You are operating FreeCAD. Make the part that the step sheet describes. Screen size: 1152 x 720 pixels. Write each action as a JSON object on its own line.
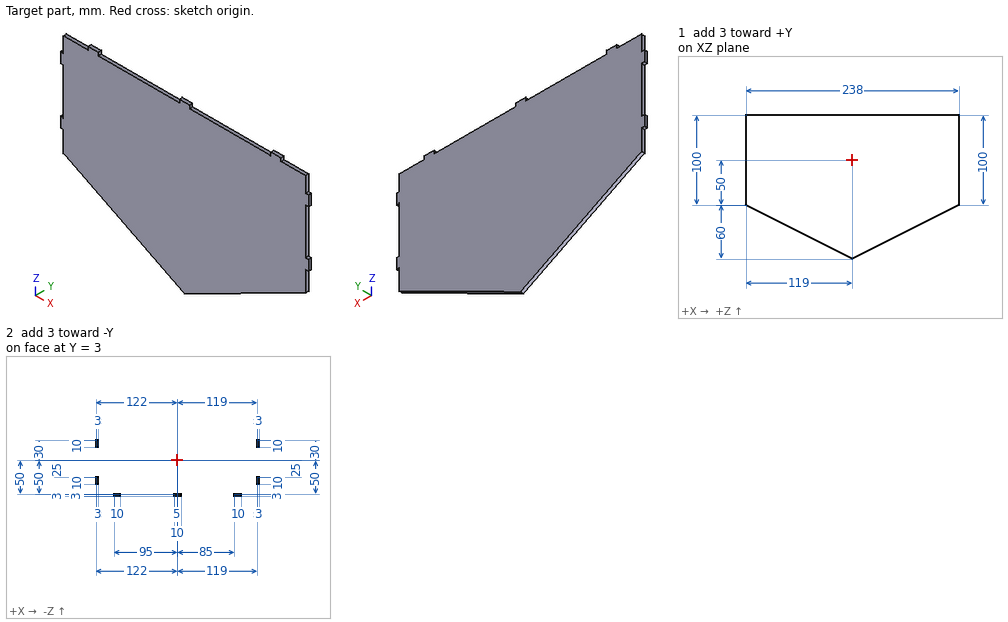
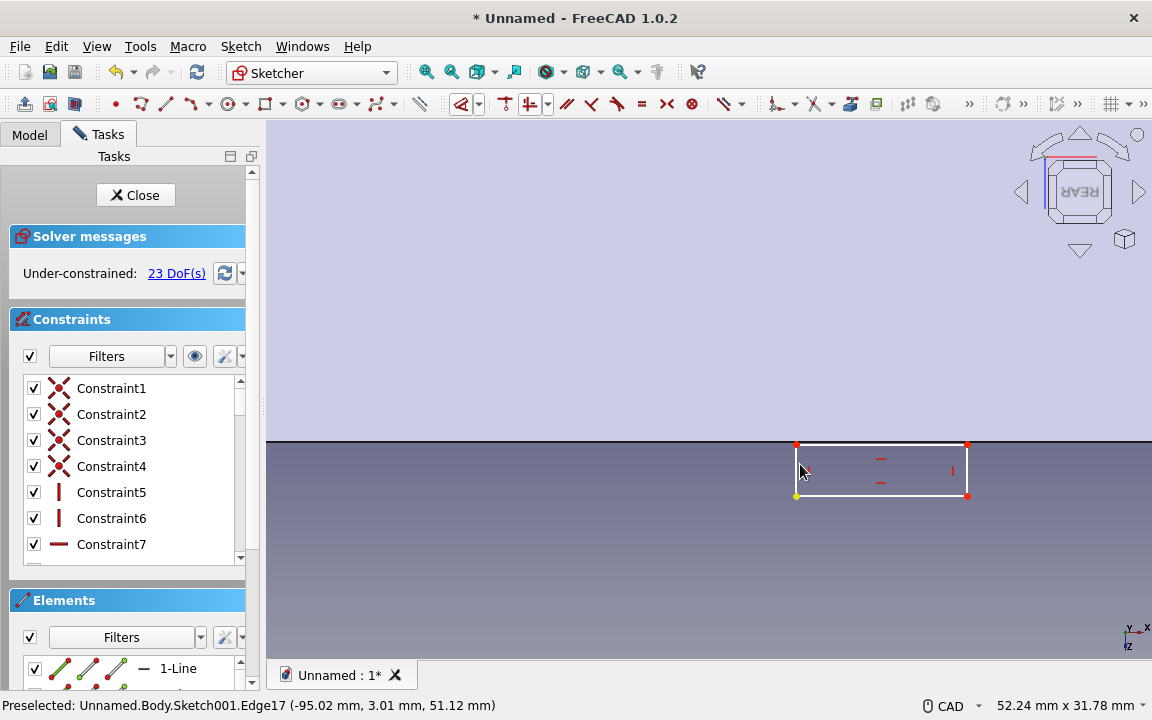
{"action": "left_click", "coordinate": [796, 460]}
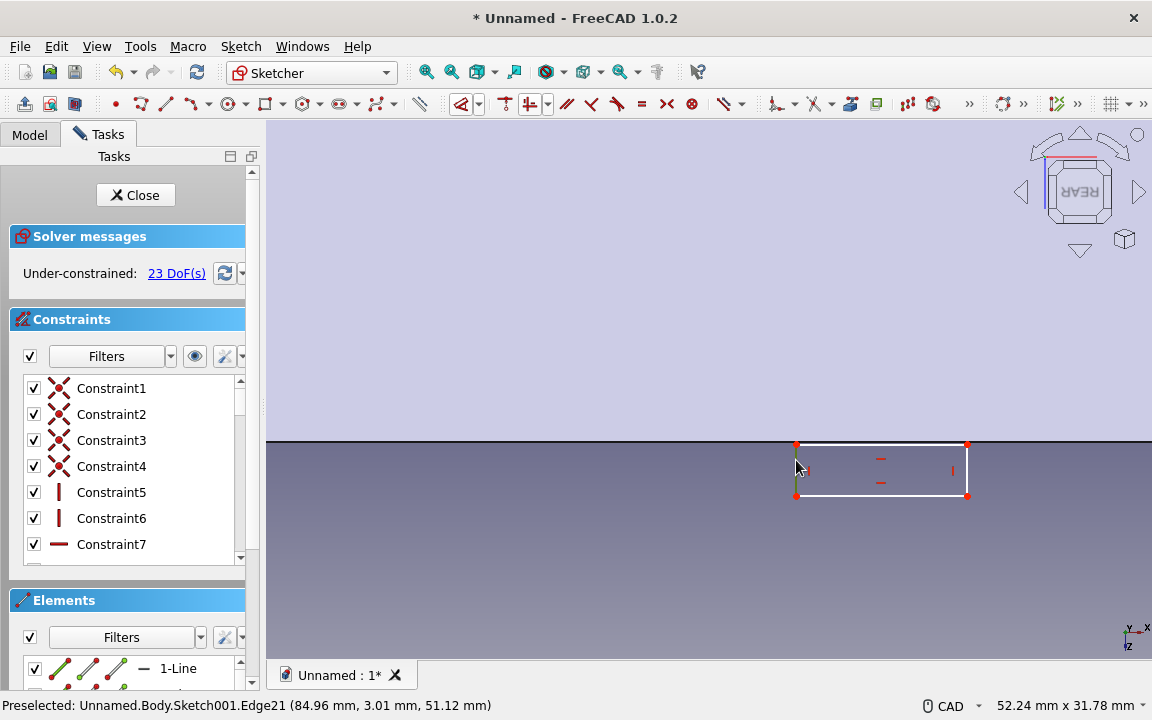
{"action": "left_click", "coordinate": [478, 104]}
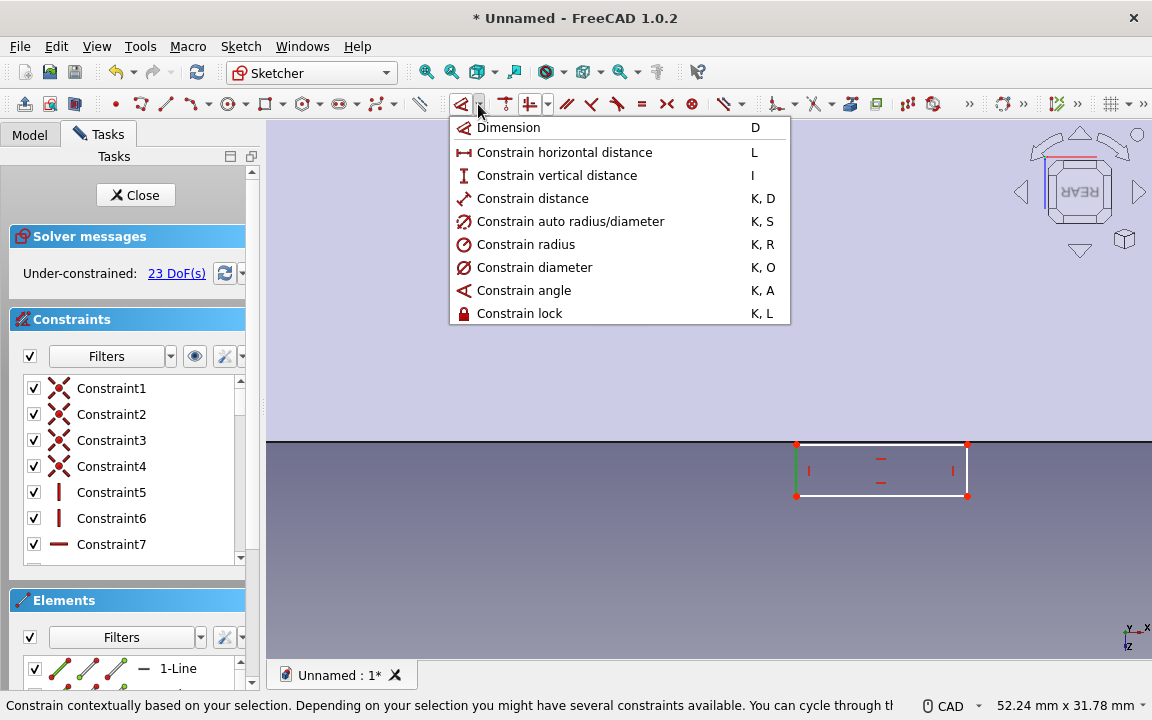
{"action": "left_click", "coordinate": [620, 176]}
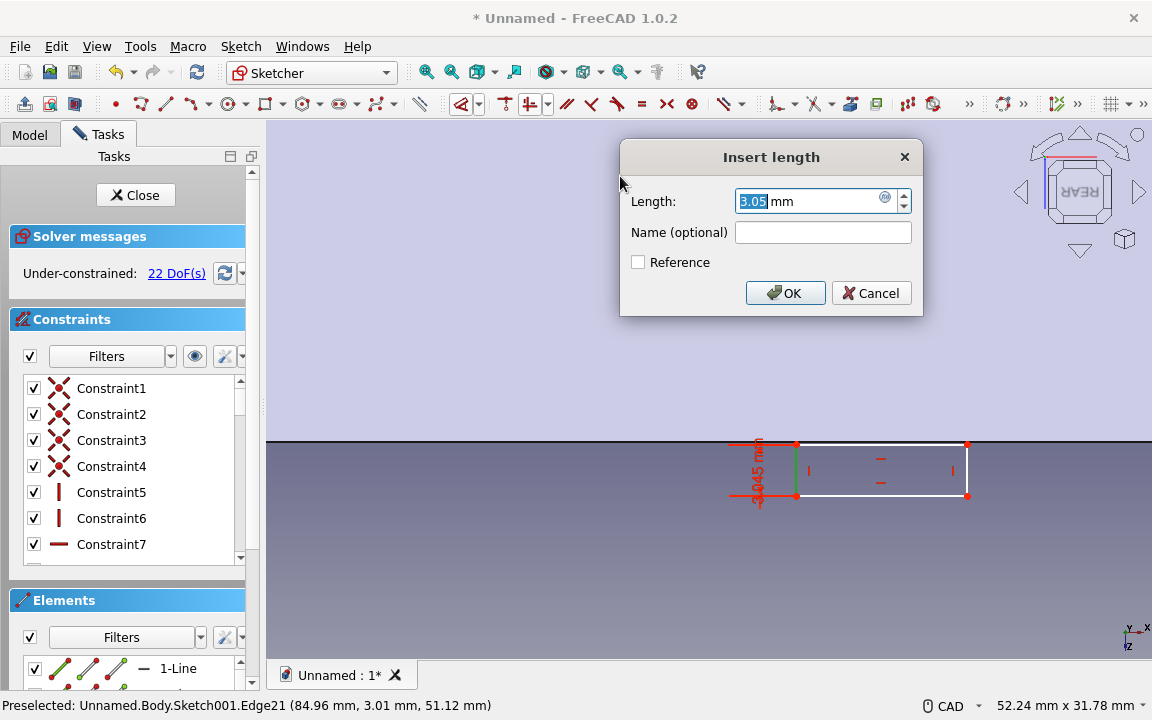
{"action": "type", "text": "3"}
{"action": "key", "text": "Return"}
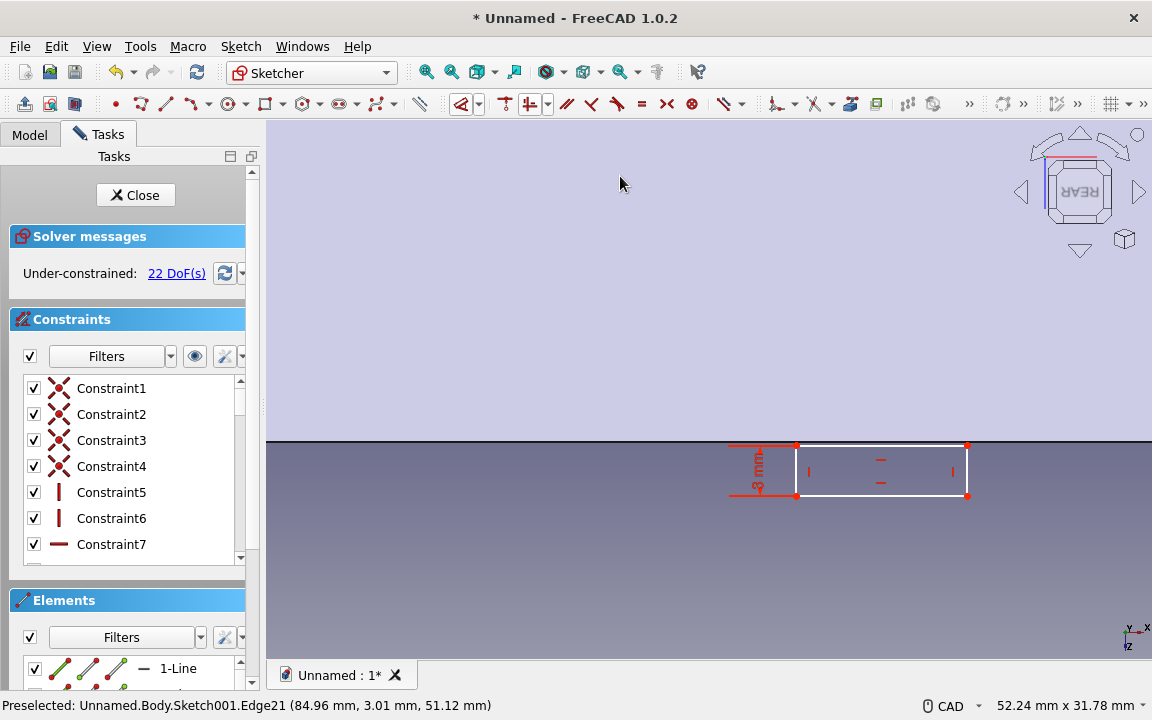
{"action": "scroll", "coordinate": [801, 464], "scroll_direction": "down", "scroll_amount": 11}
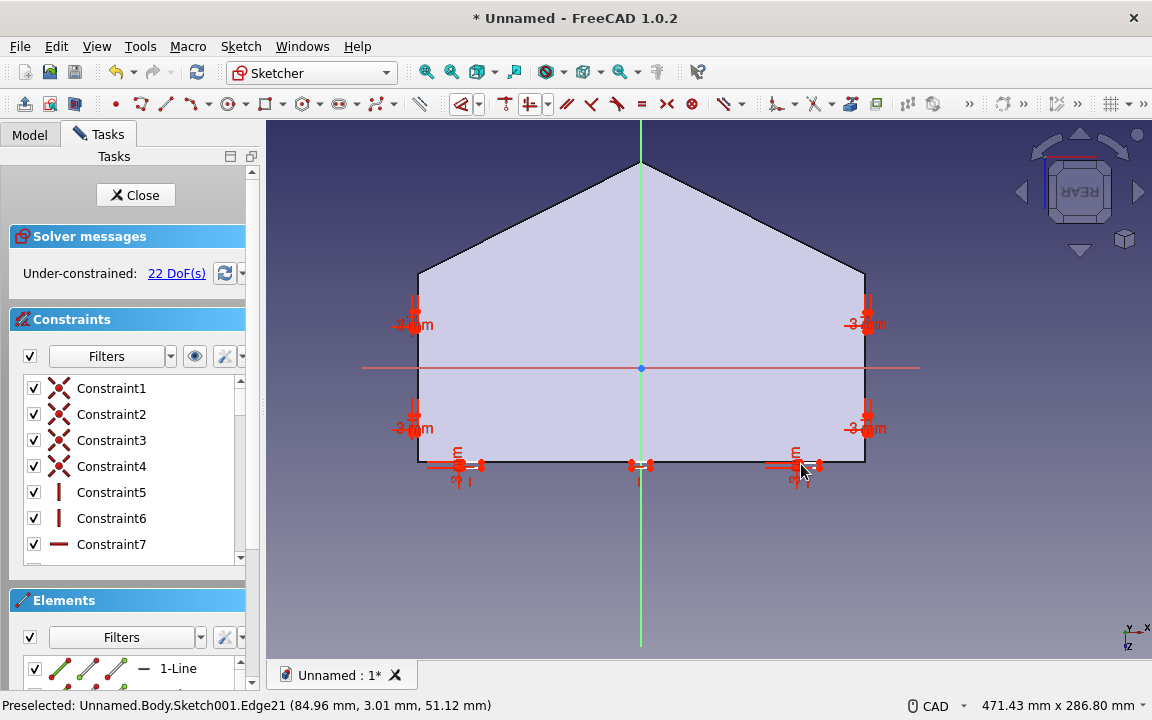
{"action": "scroll", "coordinate": [632, 464], "scroll_direction": "up", "scroll_amount": 11}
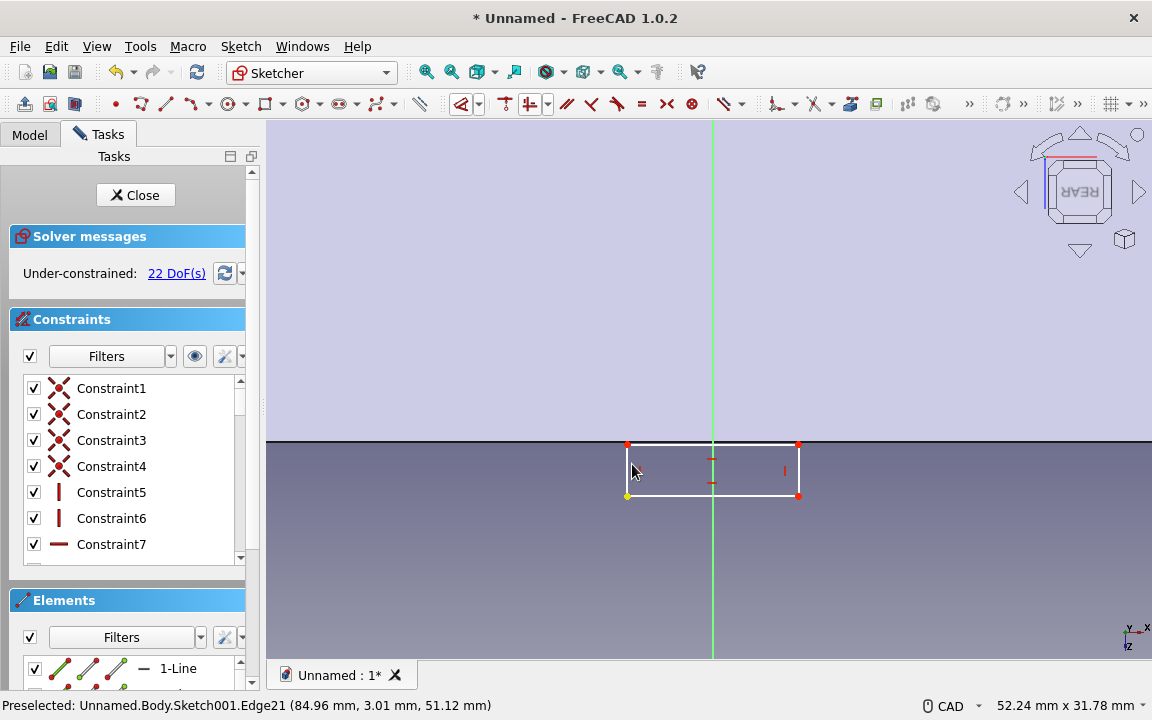
{"action": "left_click", "coordinate": [627, 460]}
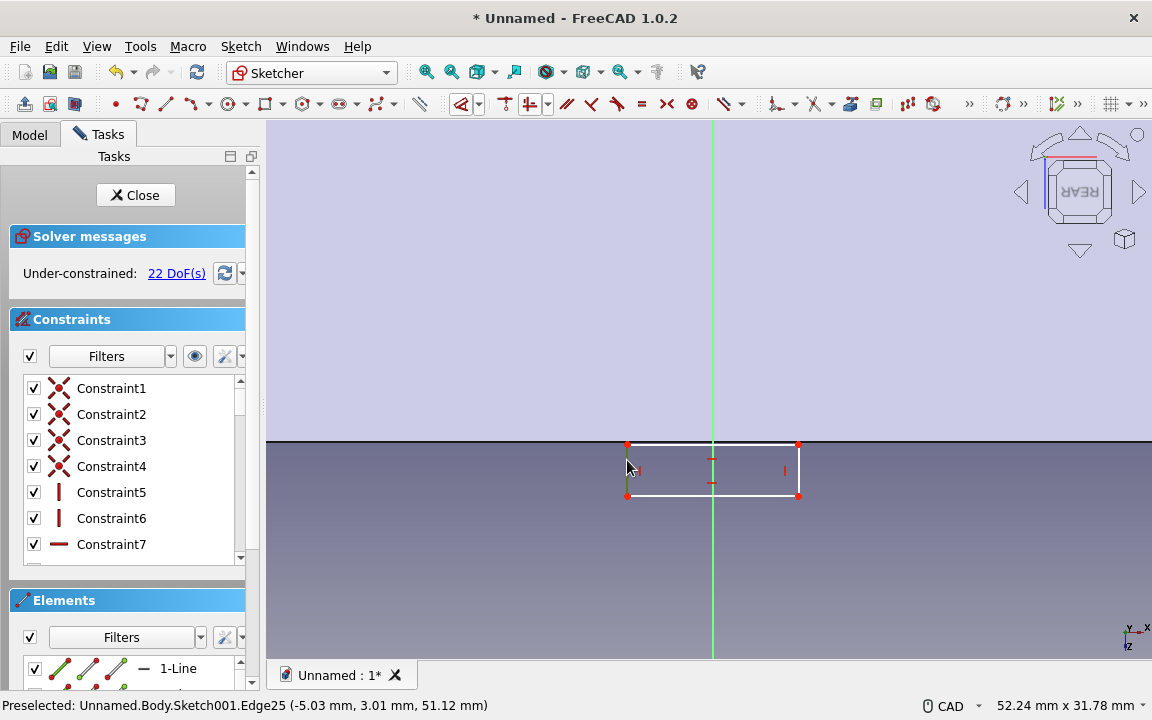
{"action": "key", "text": "i"}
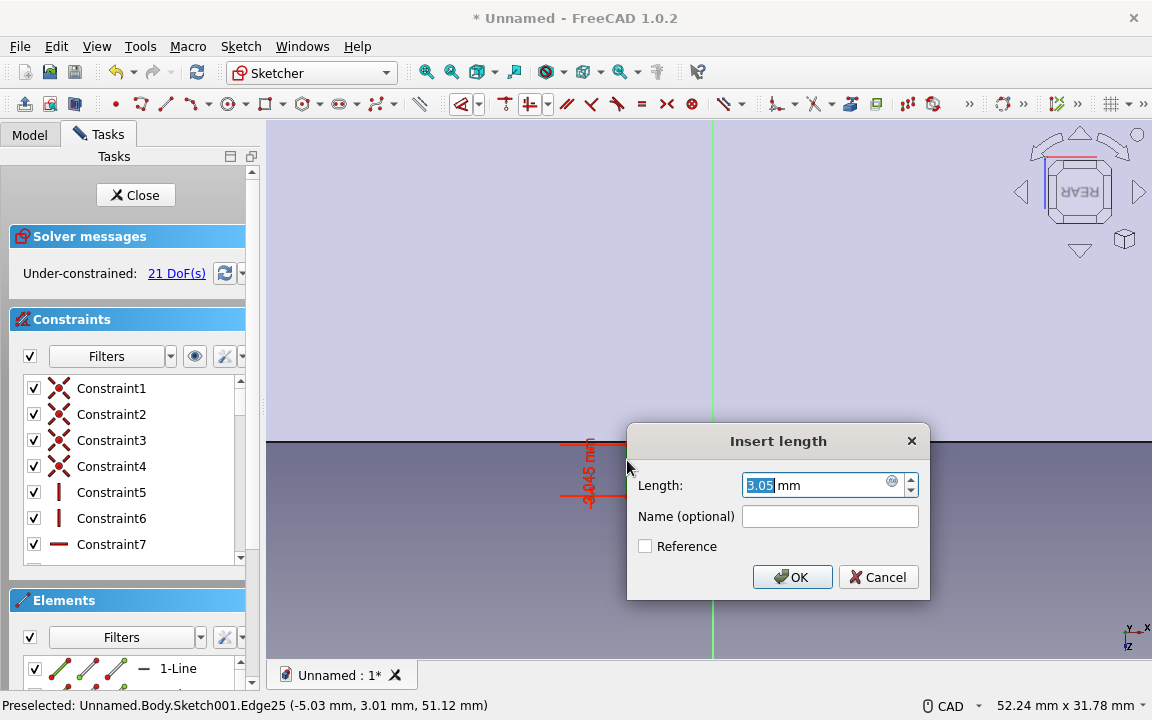
{"action": "type", "text": "3"}
{"action": "key", "text": "Return"}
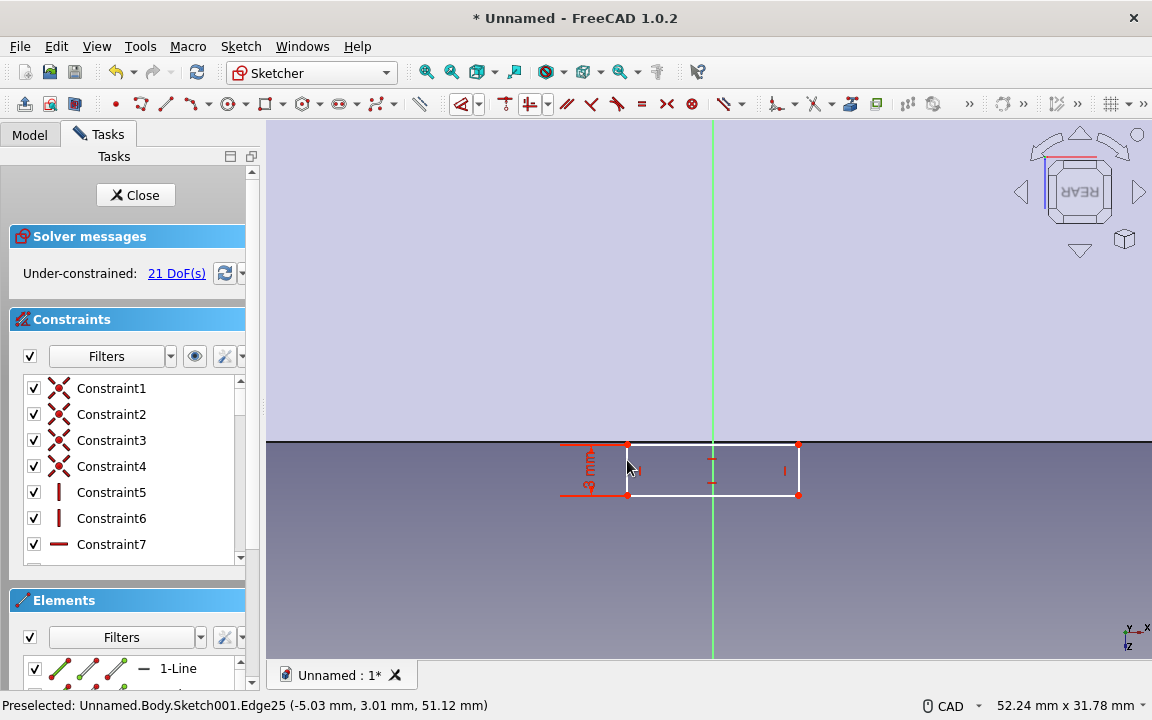
{"action": "scroll", "coordinate": [632, 464], "scroll_direction": "down", "scroll_amount": 11}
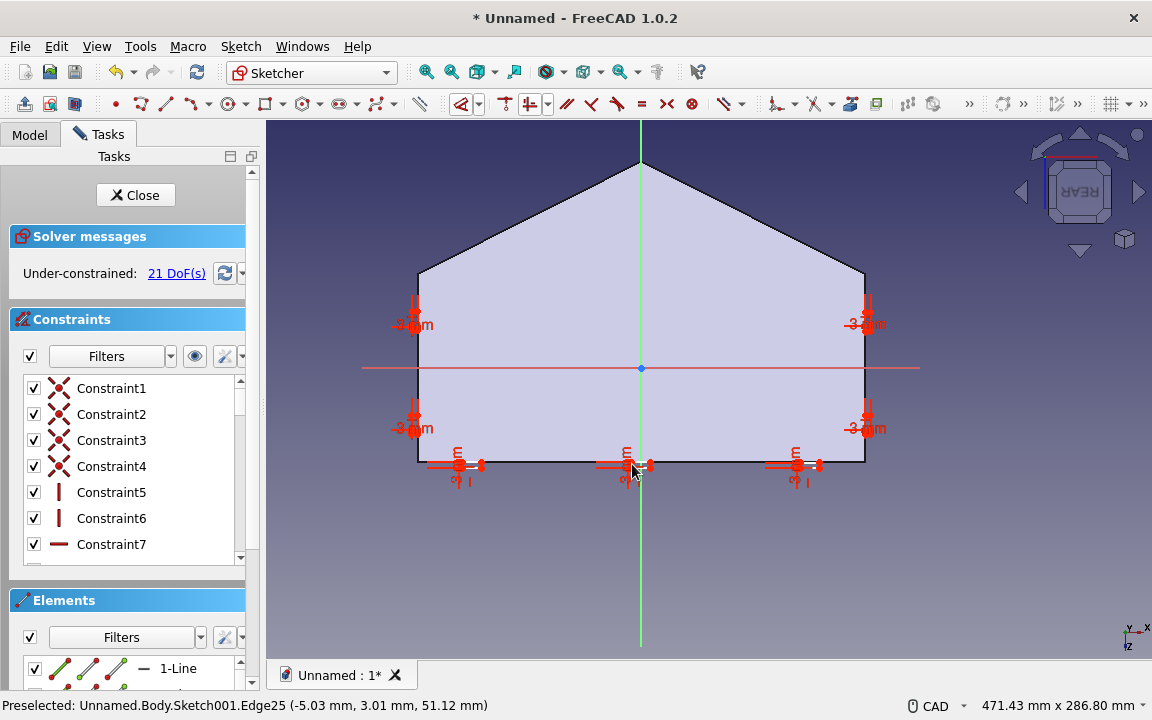
{"action": "scroll", "coordinate": [865, 318], "scroll_direction": "up", "scroll_amount": 5}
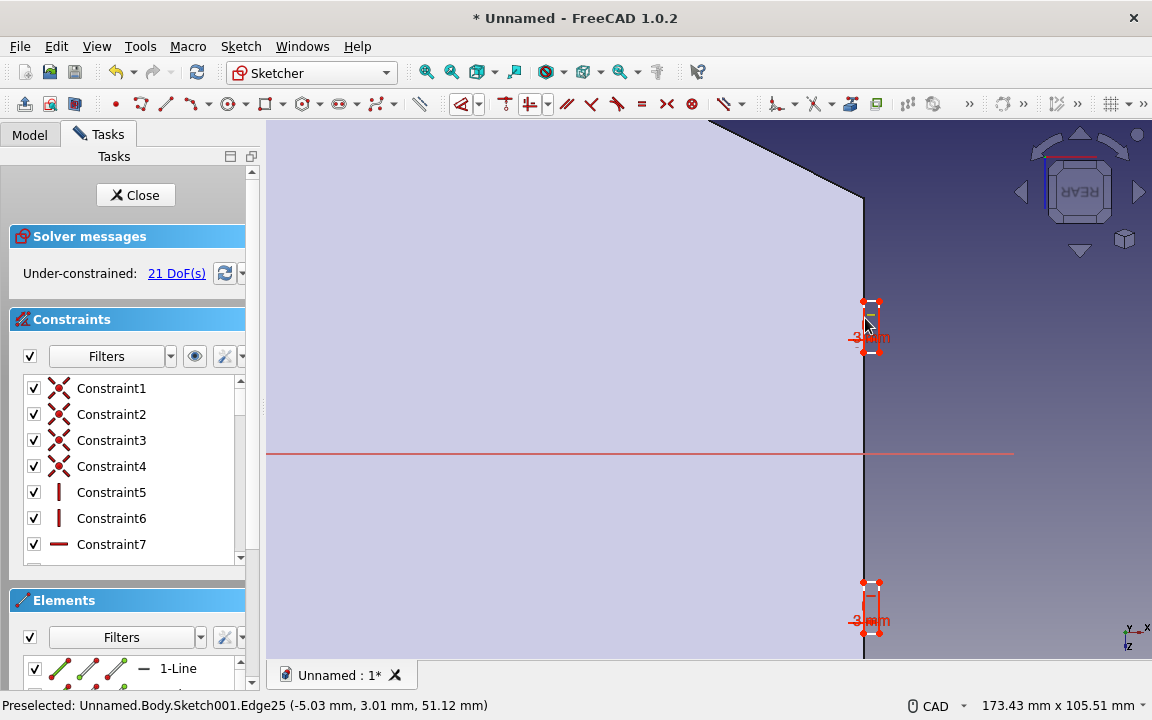
{"action": "left_click", "coordinate": [864, 317]}